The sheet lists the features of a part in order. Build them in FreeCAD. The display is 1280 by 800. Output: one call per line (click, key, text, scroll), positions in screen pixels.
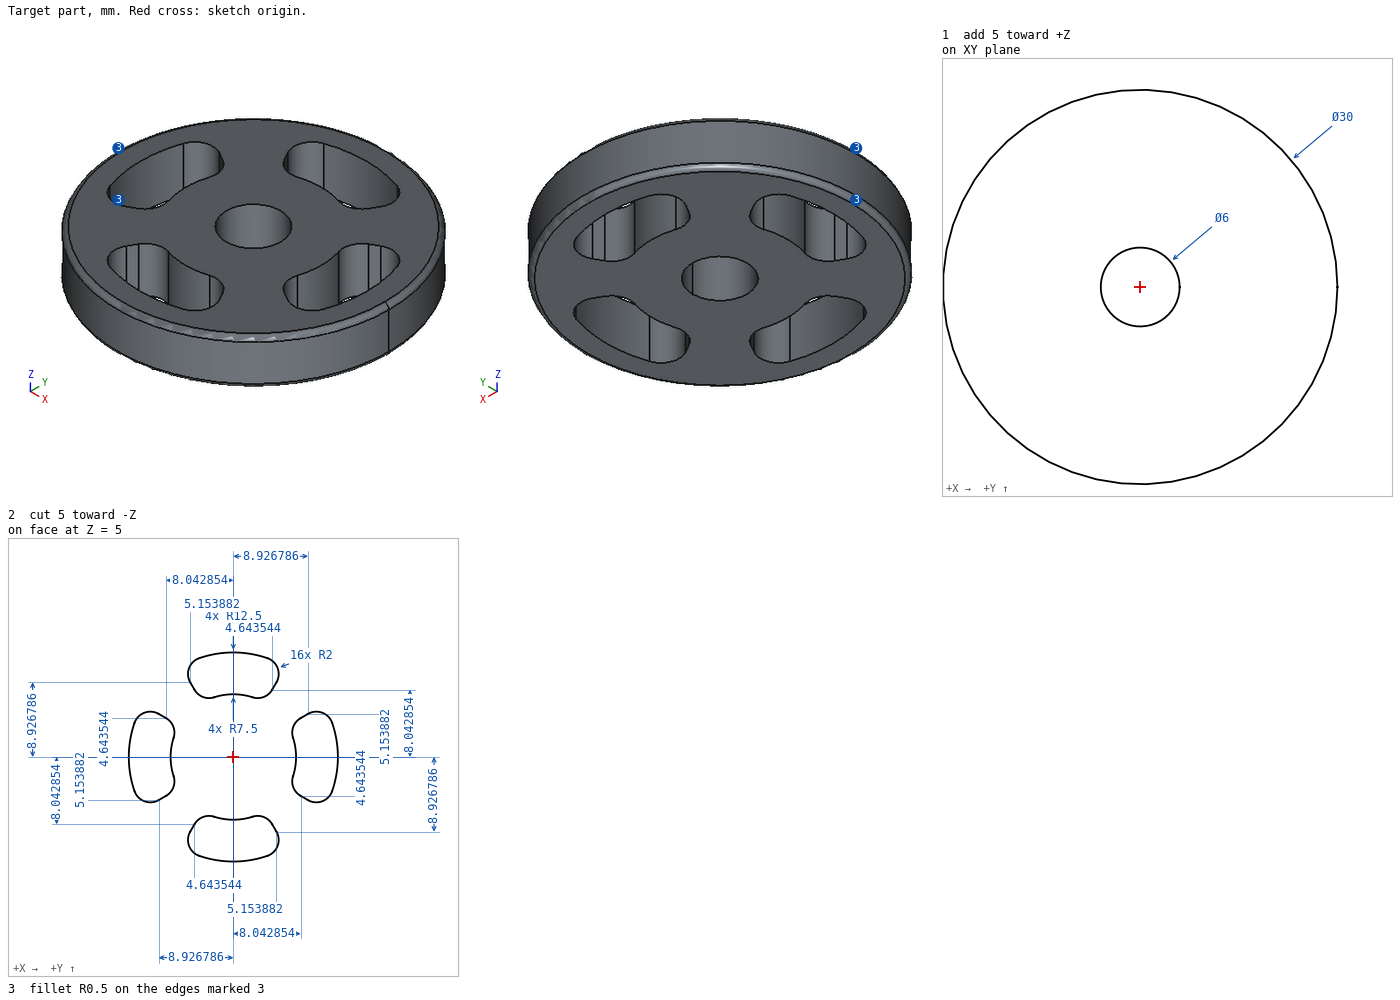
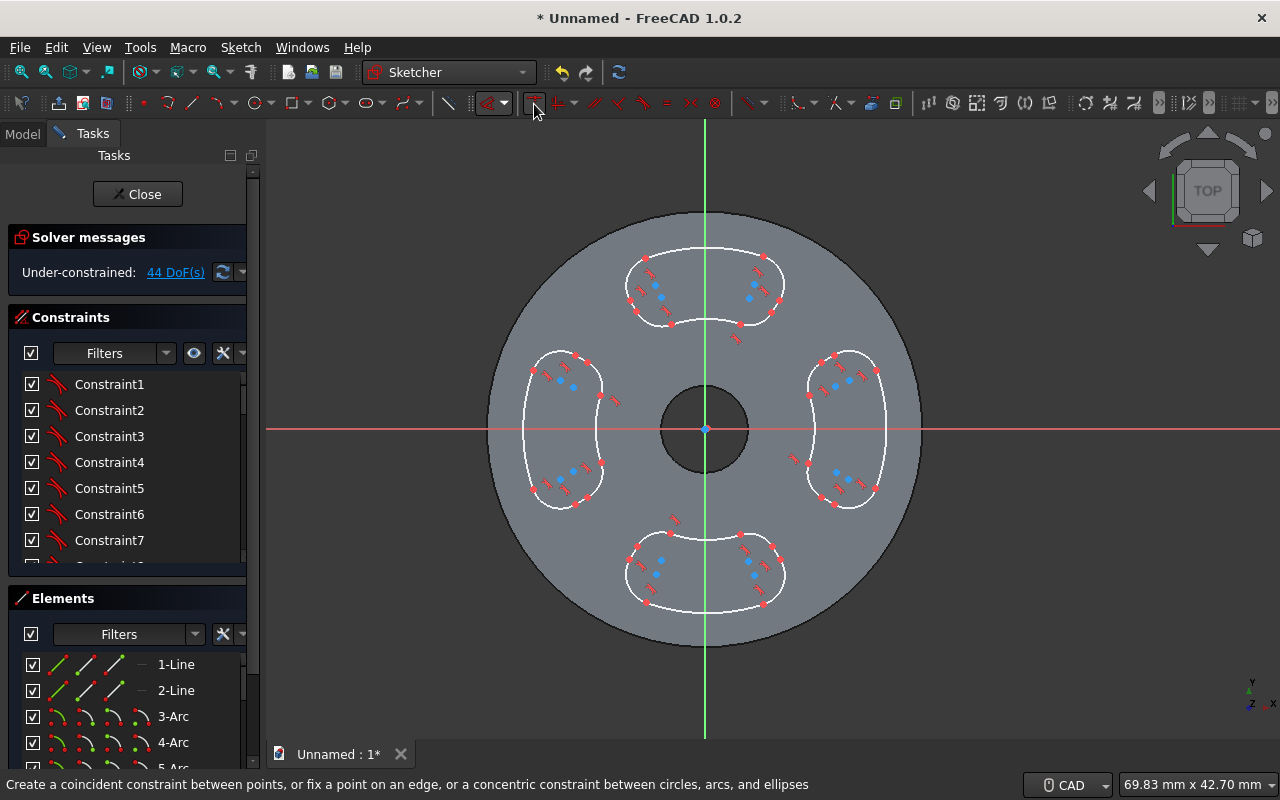
click(720, 320)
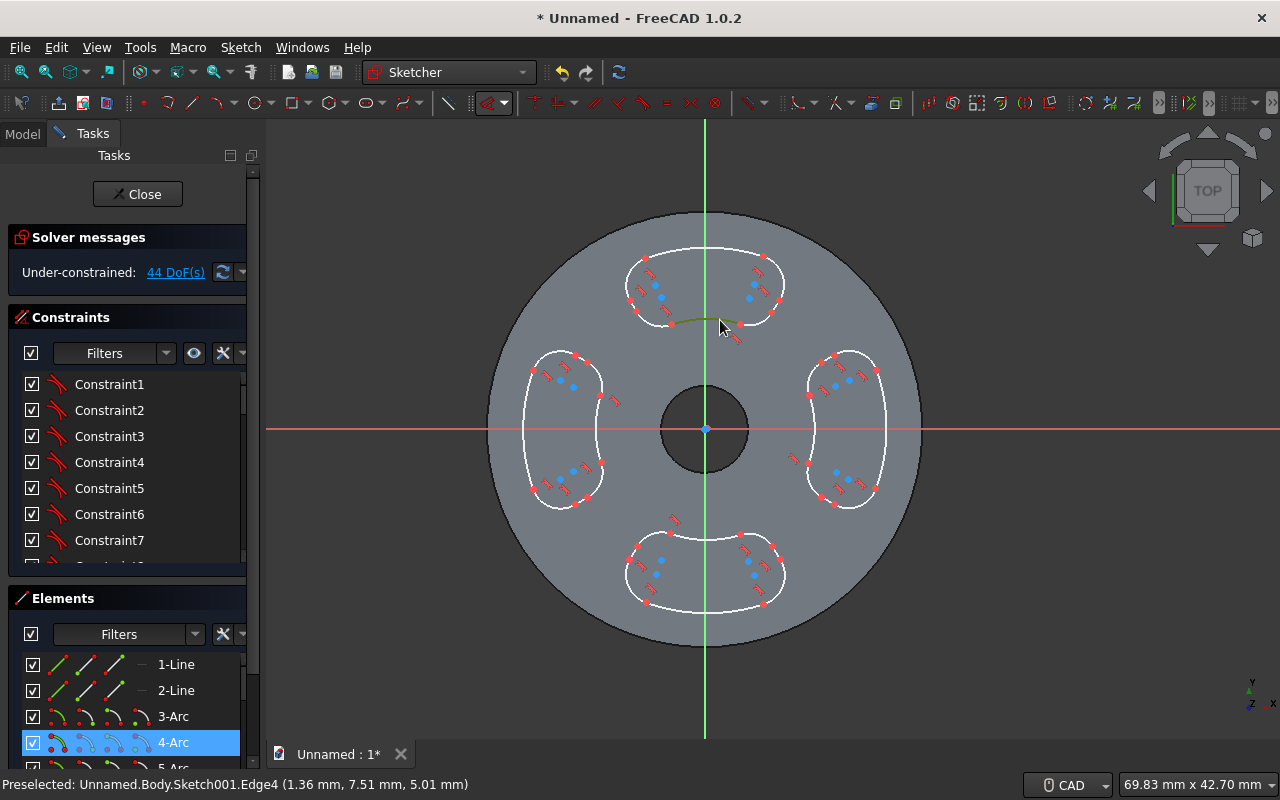
click(525, 406)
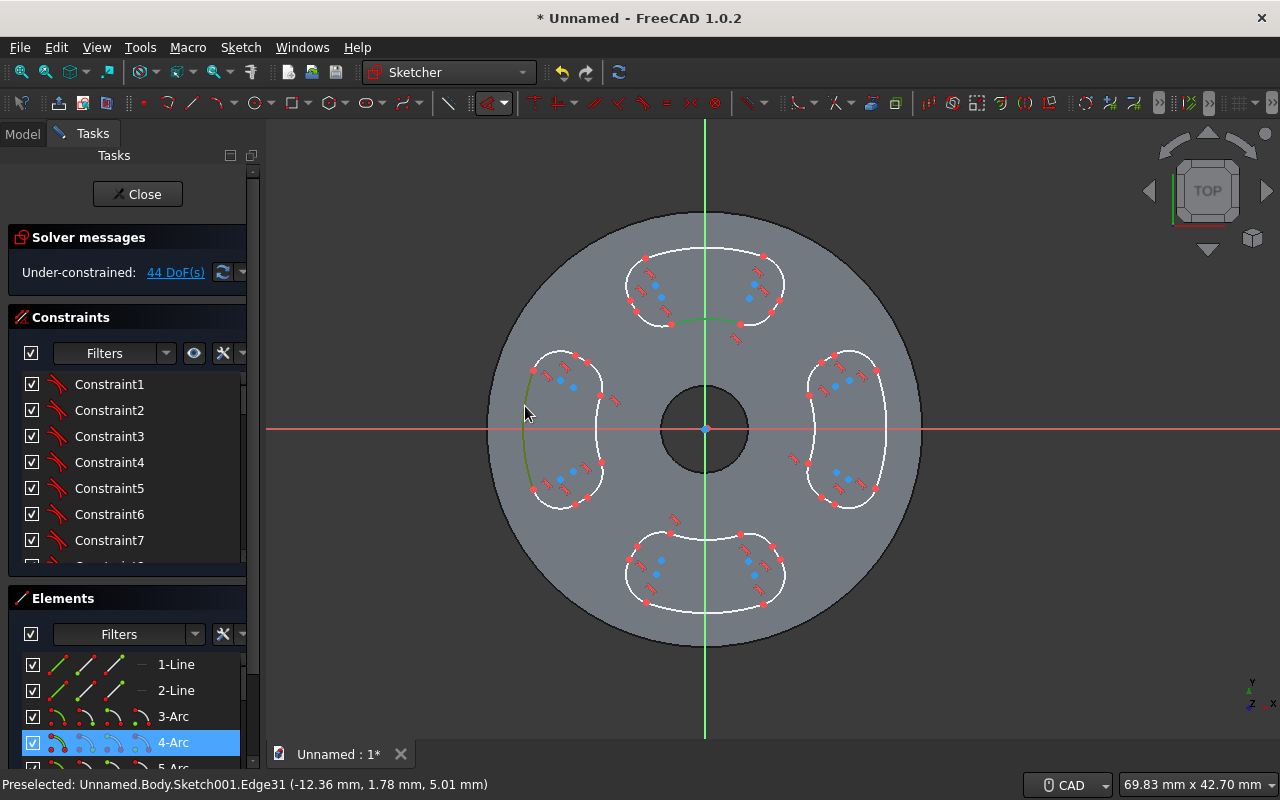
click(534, 104)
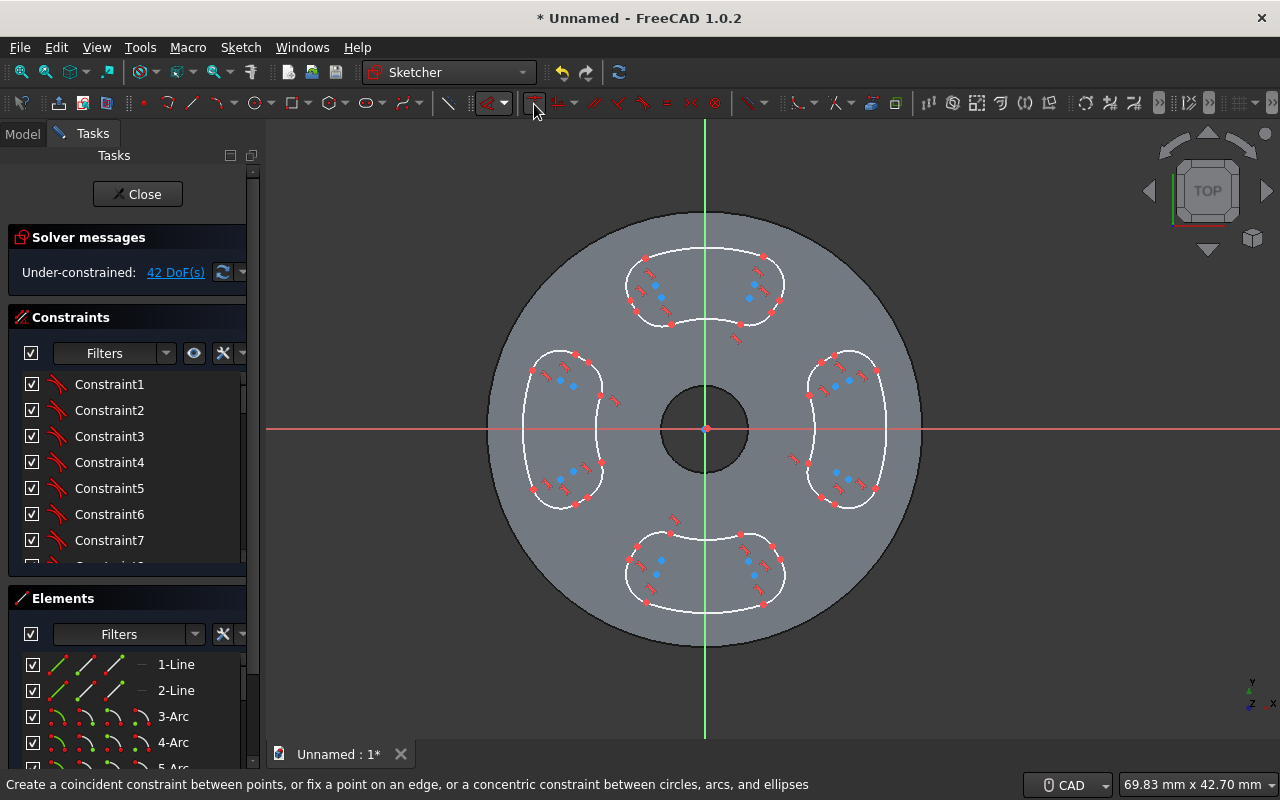
scroll(706, 429, up, 2)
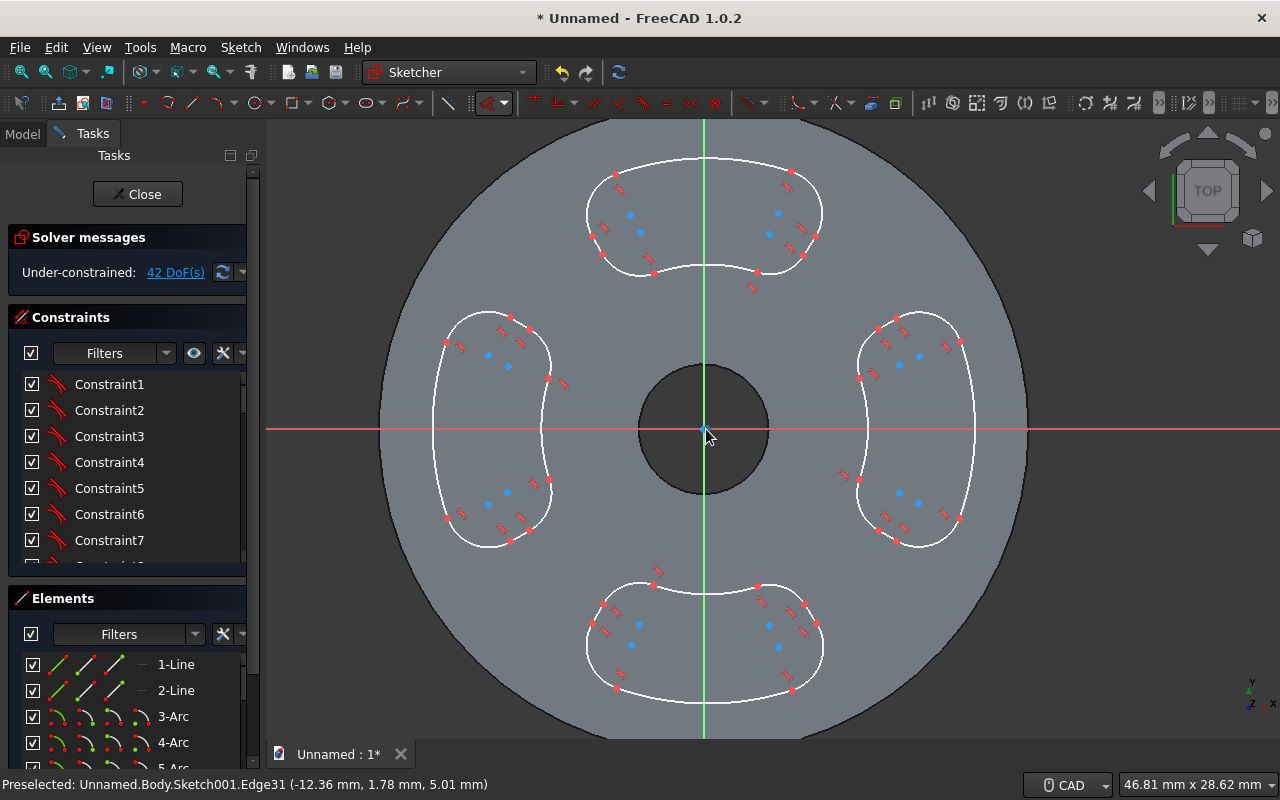
drag(694, 418, 718, 439)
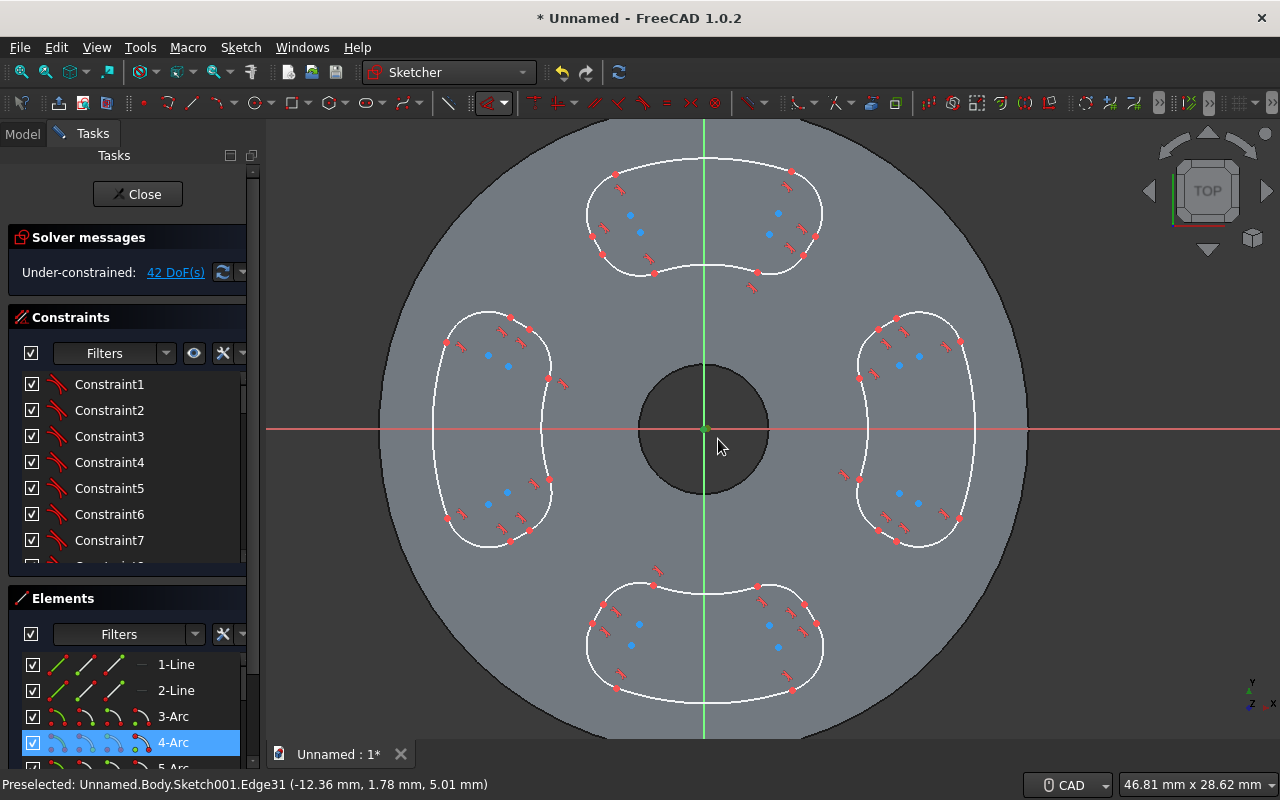
click(534, 104)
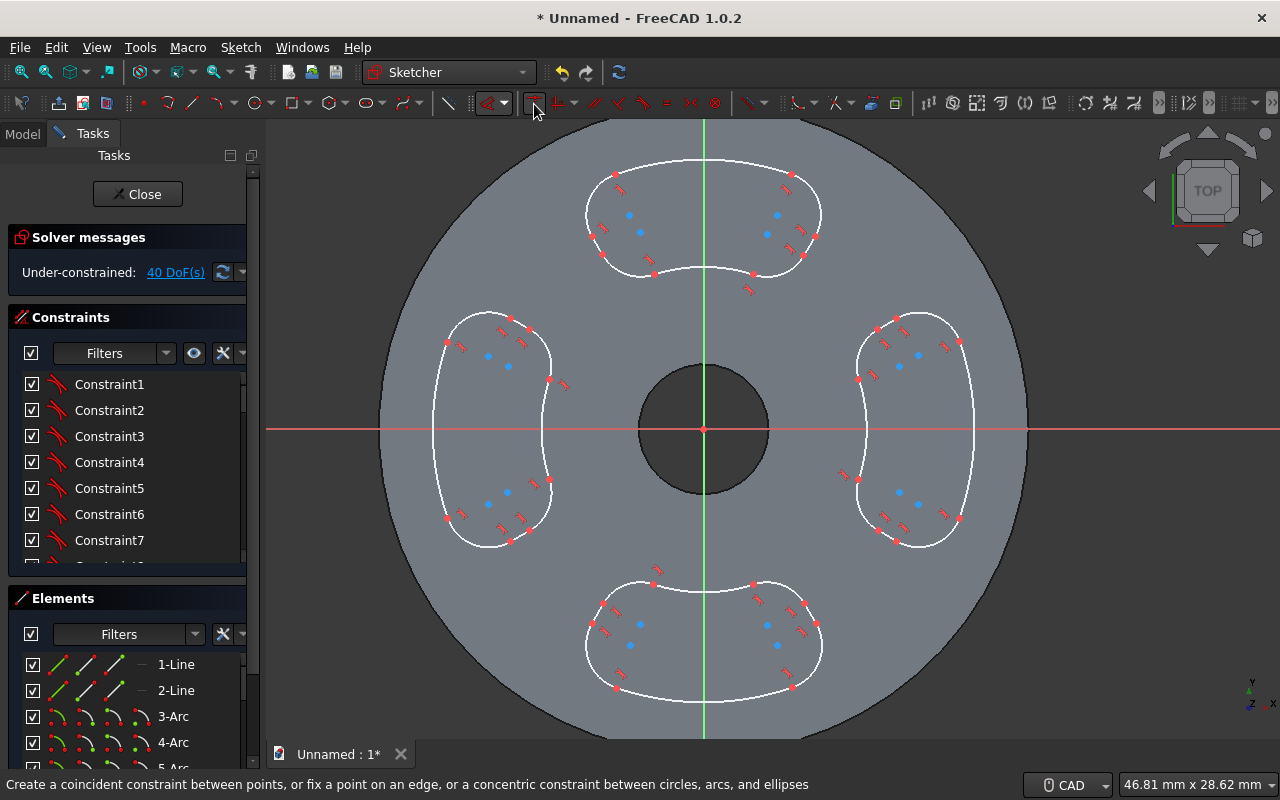
click(614, 268)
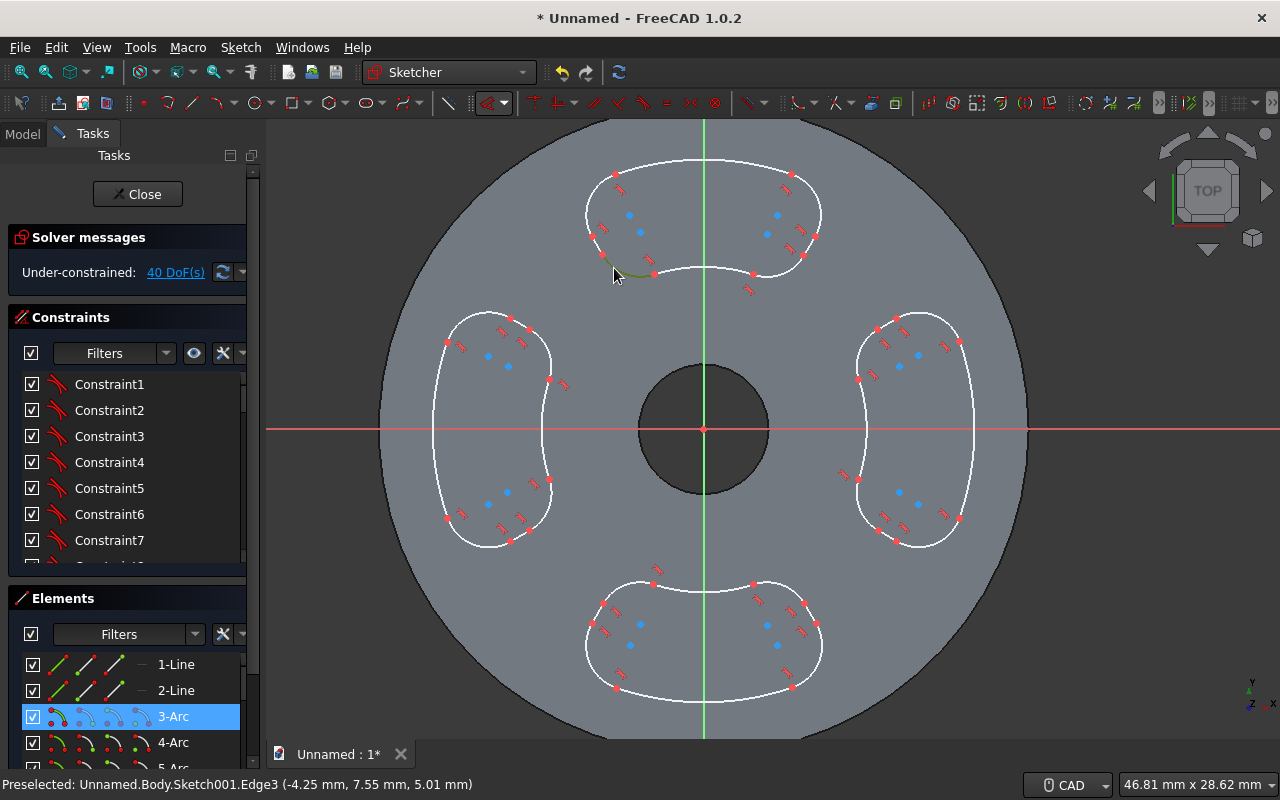
click(771, 277)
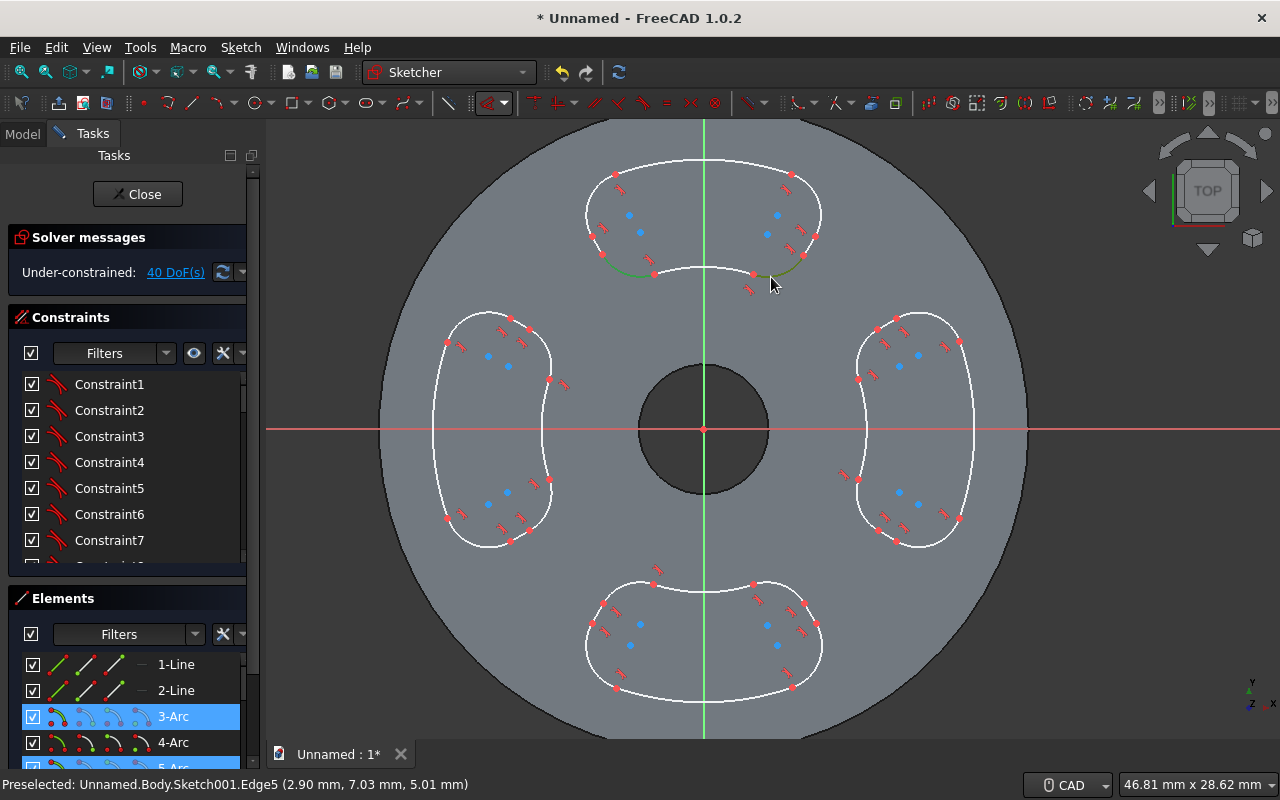
click(821, 215)